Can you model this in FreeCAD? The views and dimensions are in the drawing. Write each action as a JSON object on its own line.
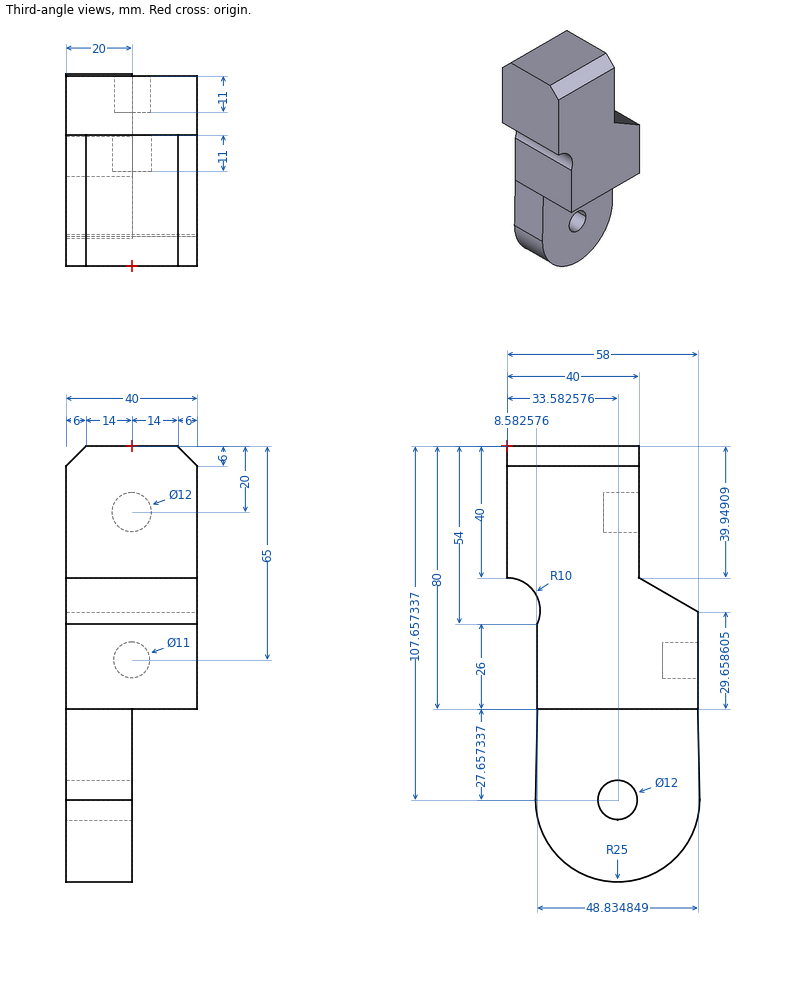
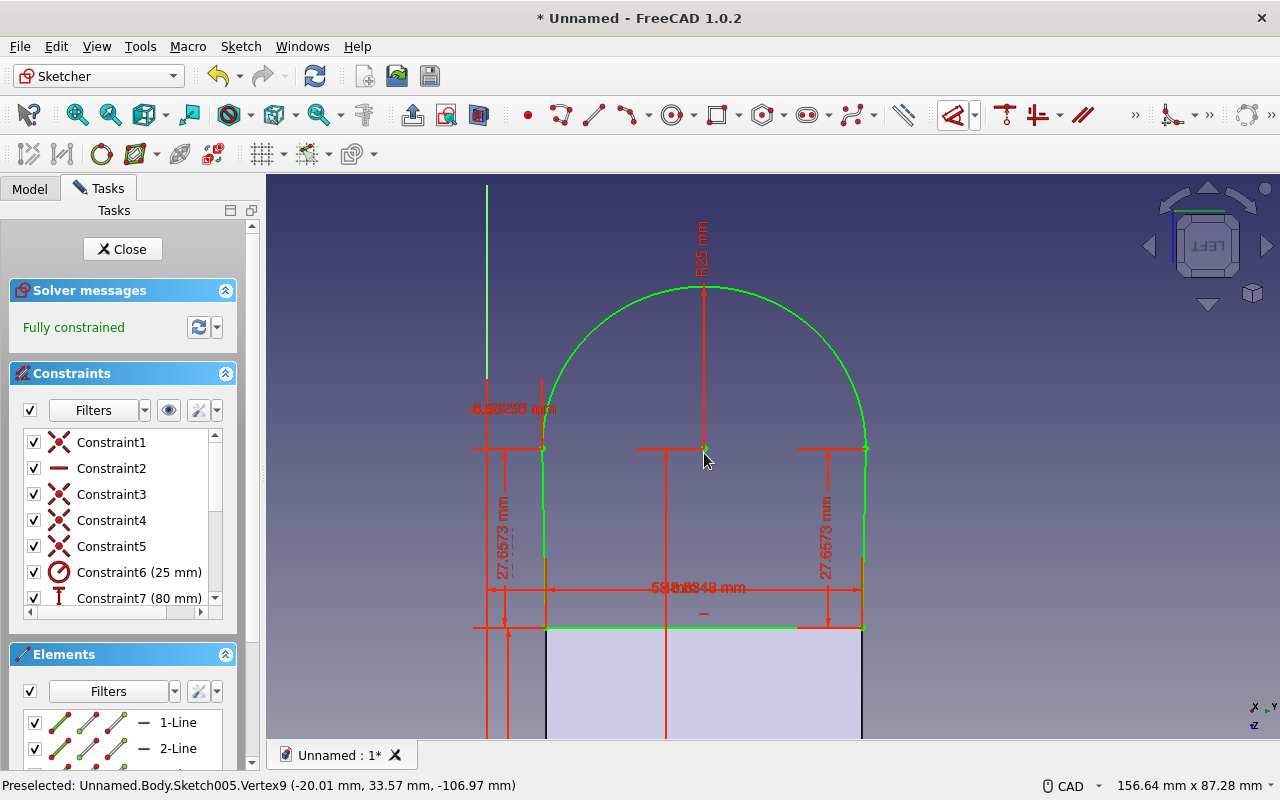
{"action": "left_click", "coordinate": [123, 249]}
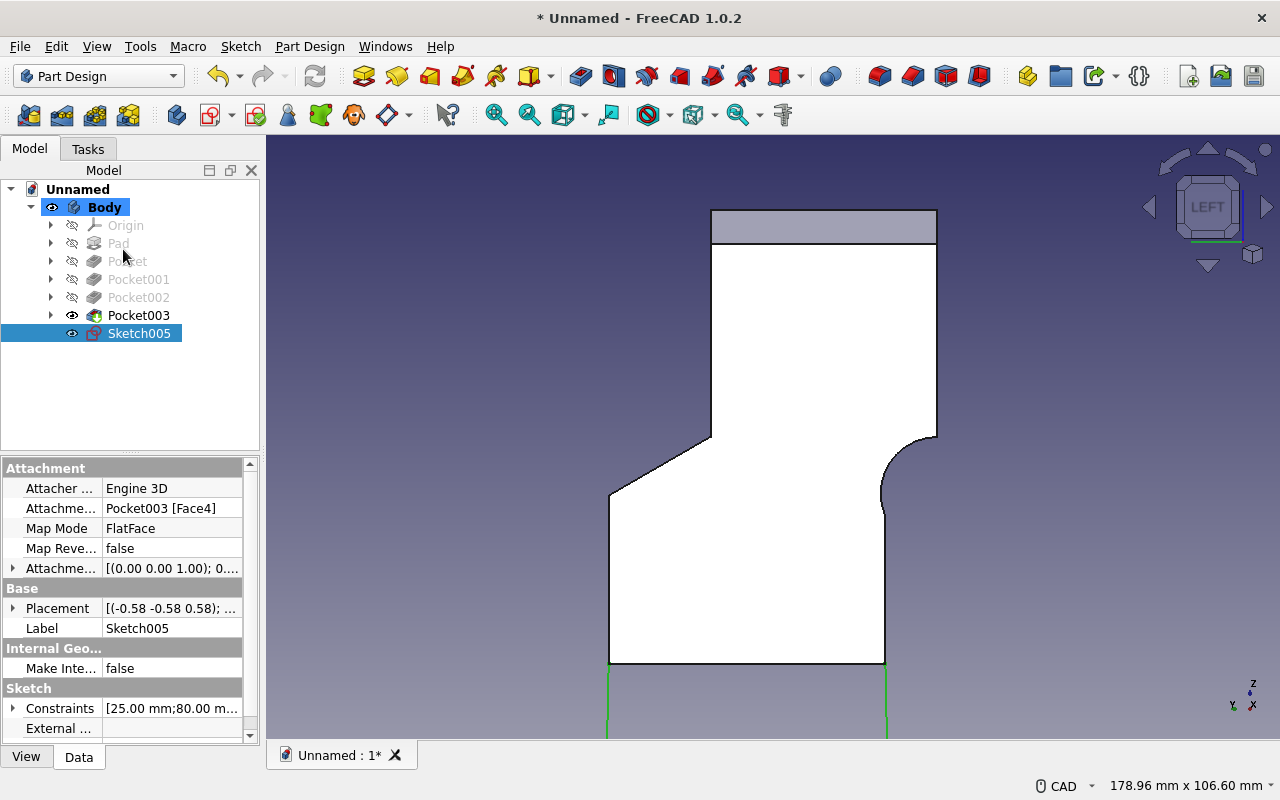
{"action": "left_click", "coordinate": [364, 76]}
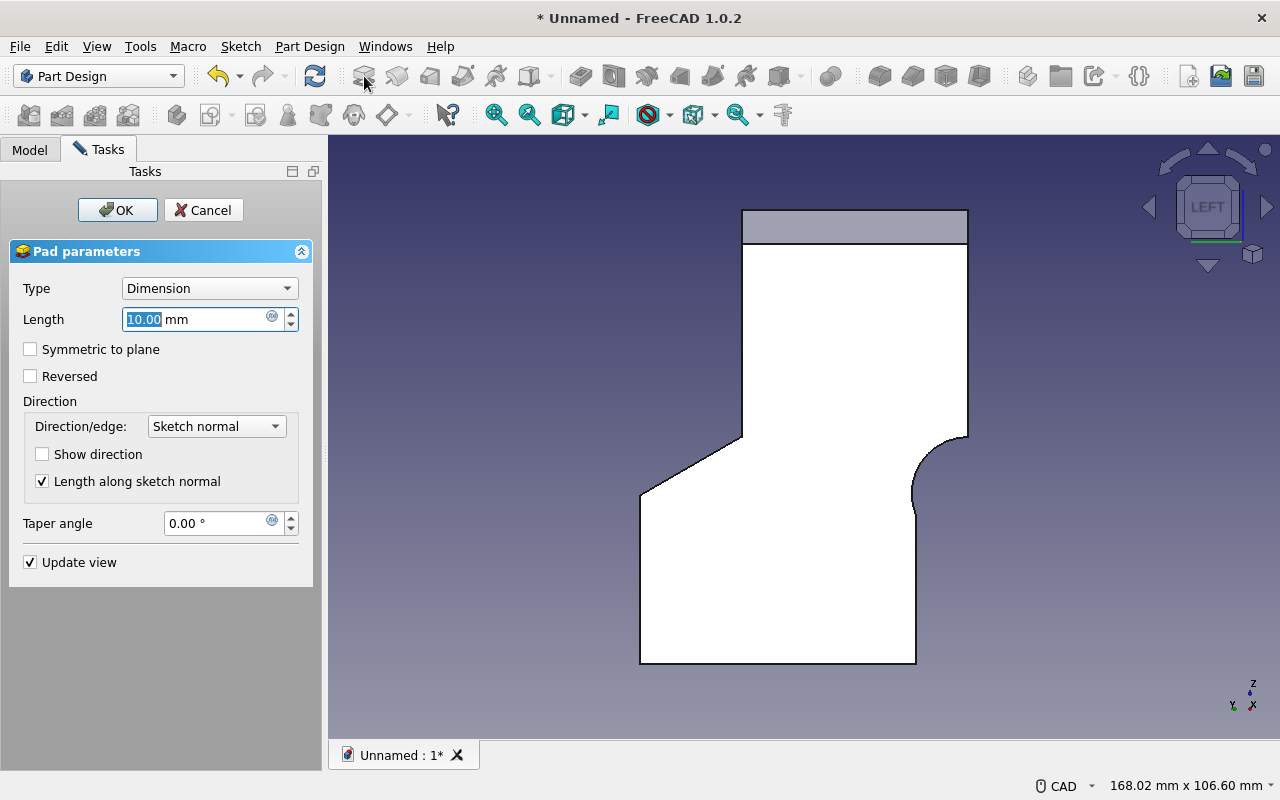
{"action": "type", "text": "20"}
{"action": "key", "text": "Tab"}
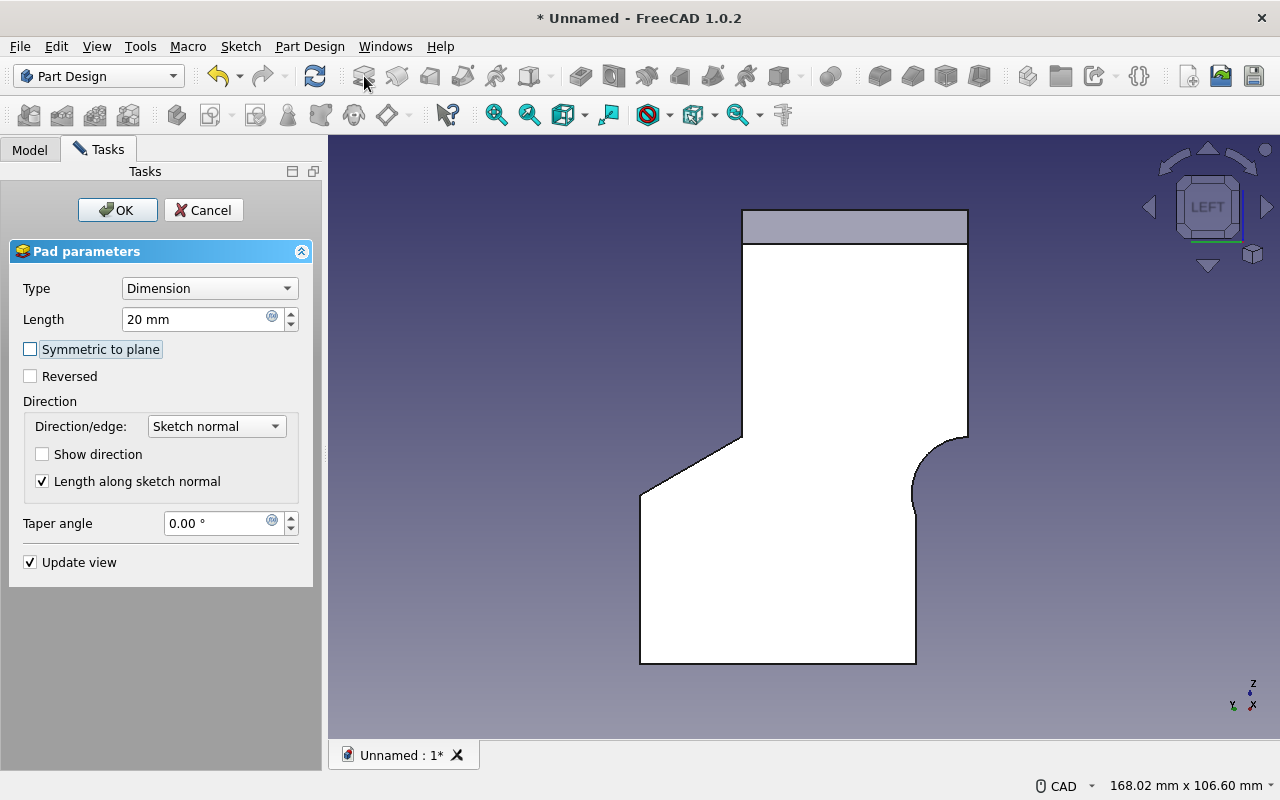
{"action": "left_click", "coordinate": [31, 376]}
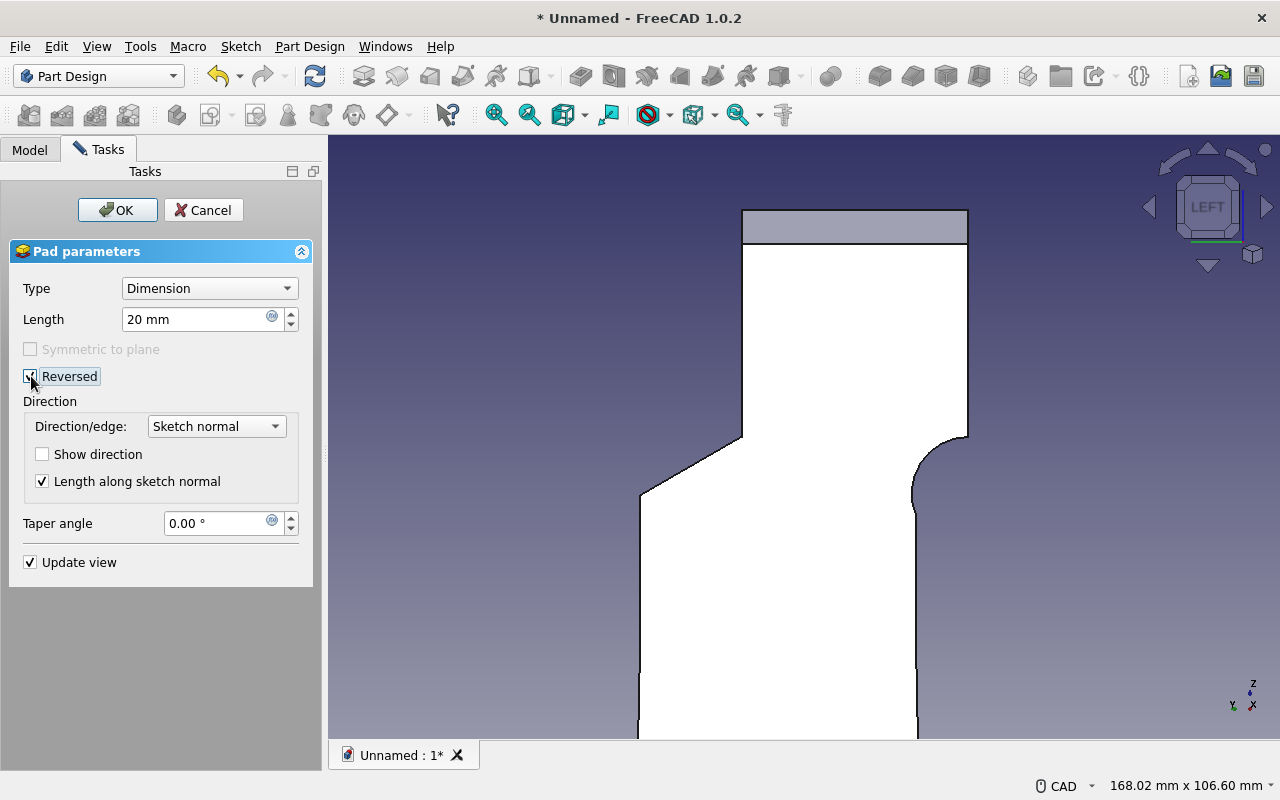
{"action": "left_click", "coordinate": [118, 210]}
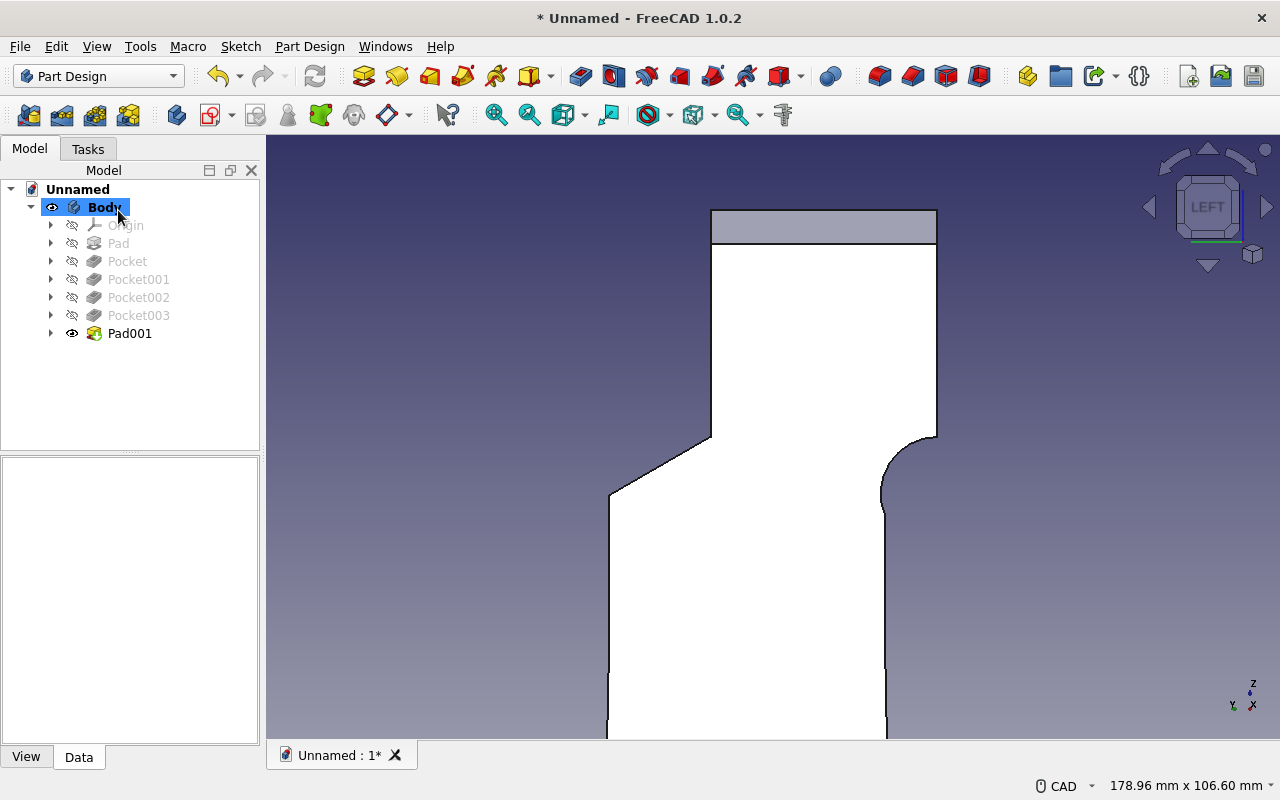
{"action": "key", "text": "v f"}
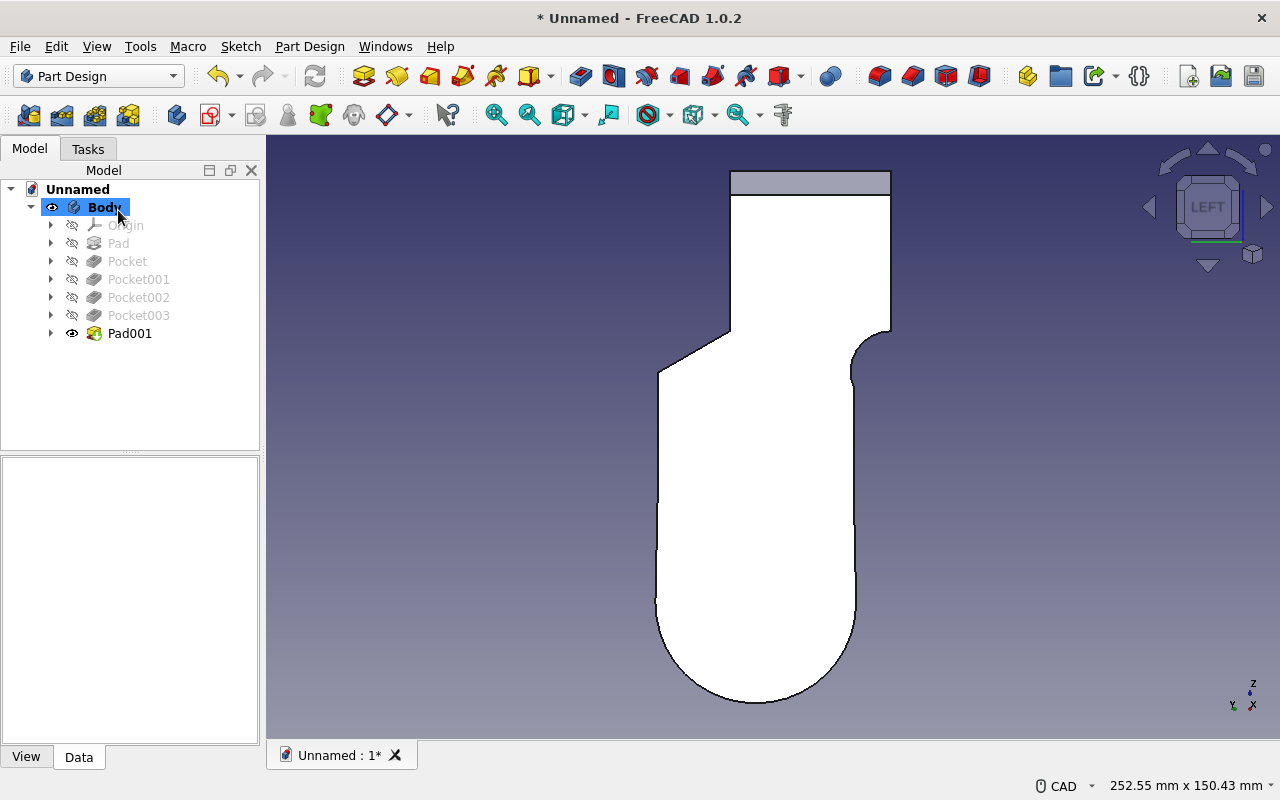
{"action": "left_click", "coordinate": [210, 116]}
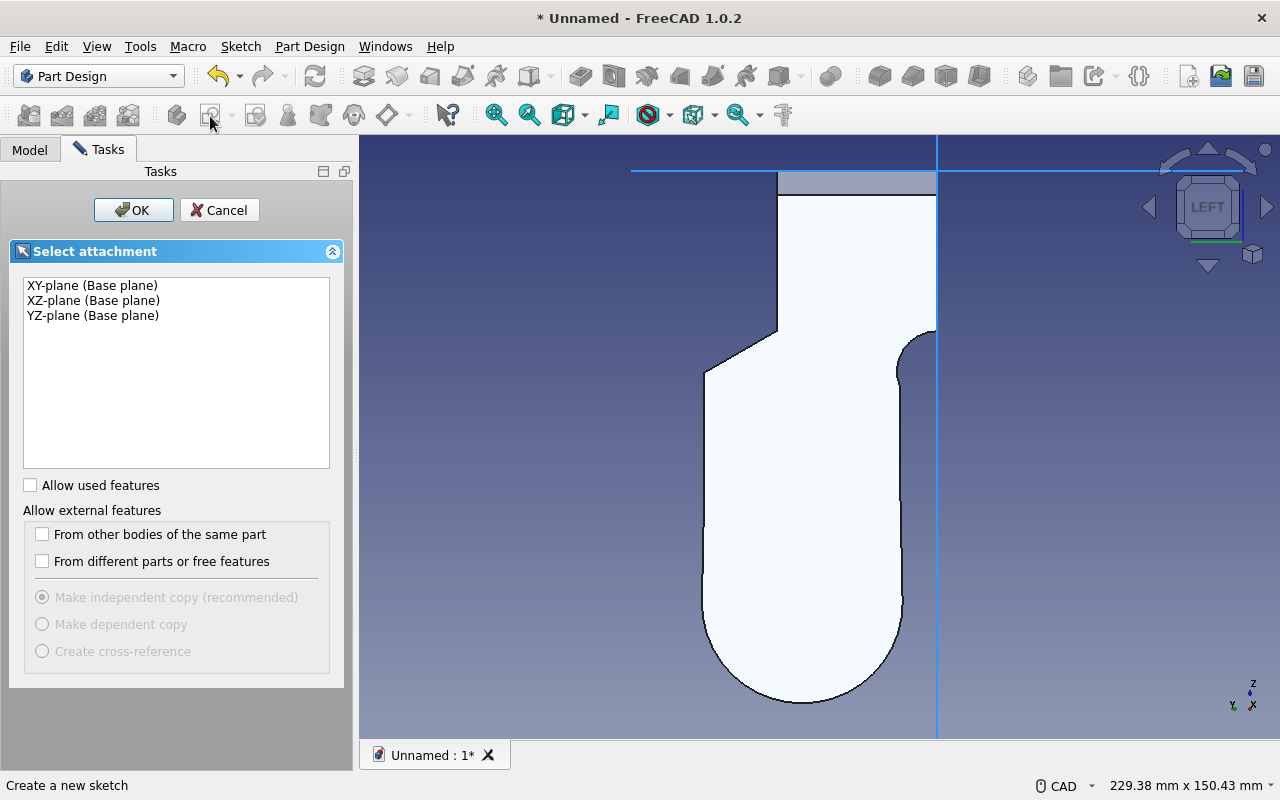
{"action": "left_click", "coordinate": [84, 316]}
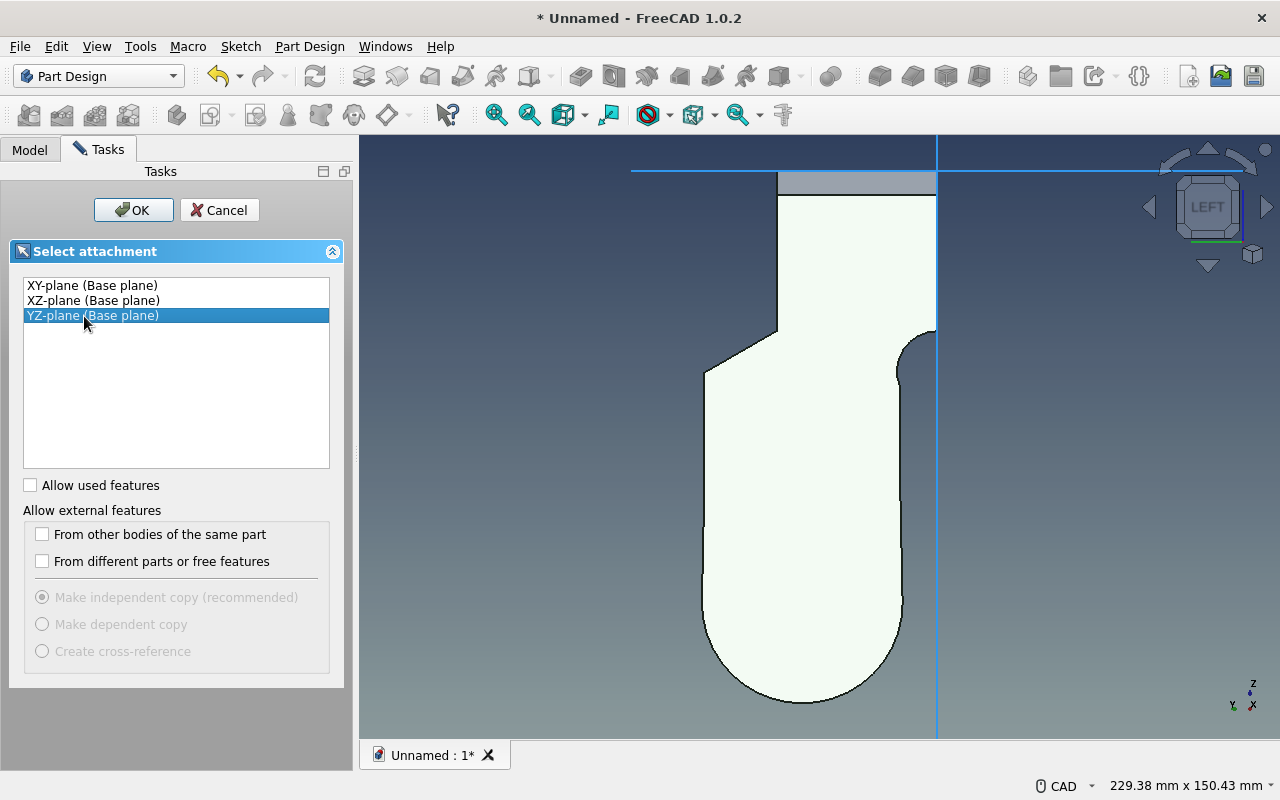
{"action": "left_click", "coordinate": [134, 210]}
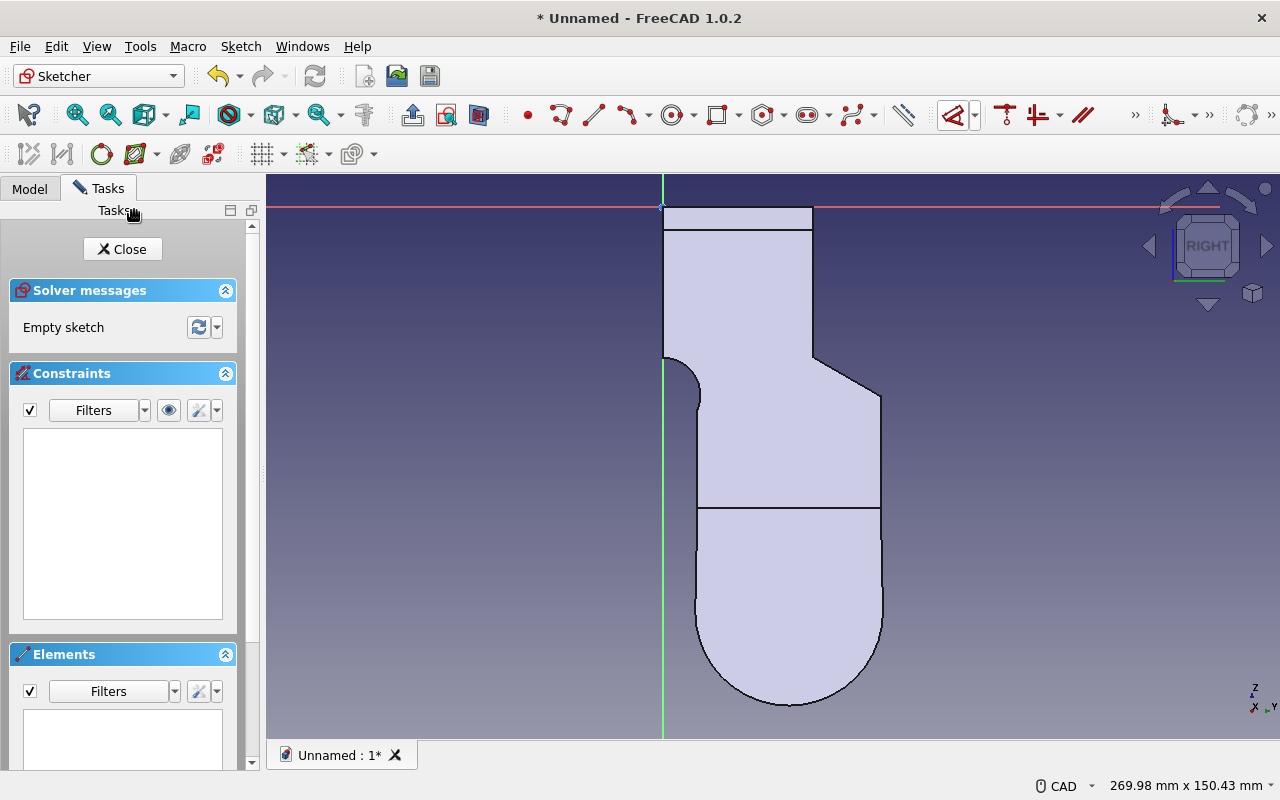
{"action": "key", "text": "q s"}